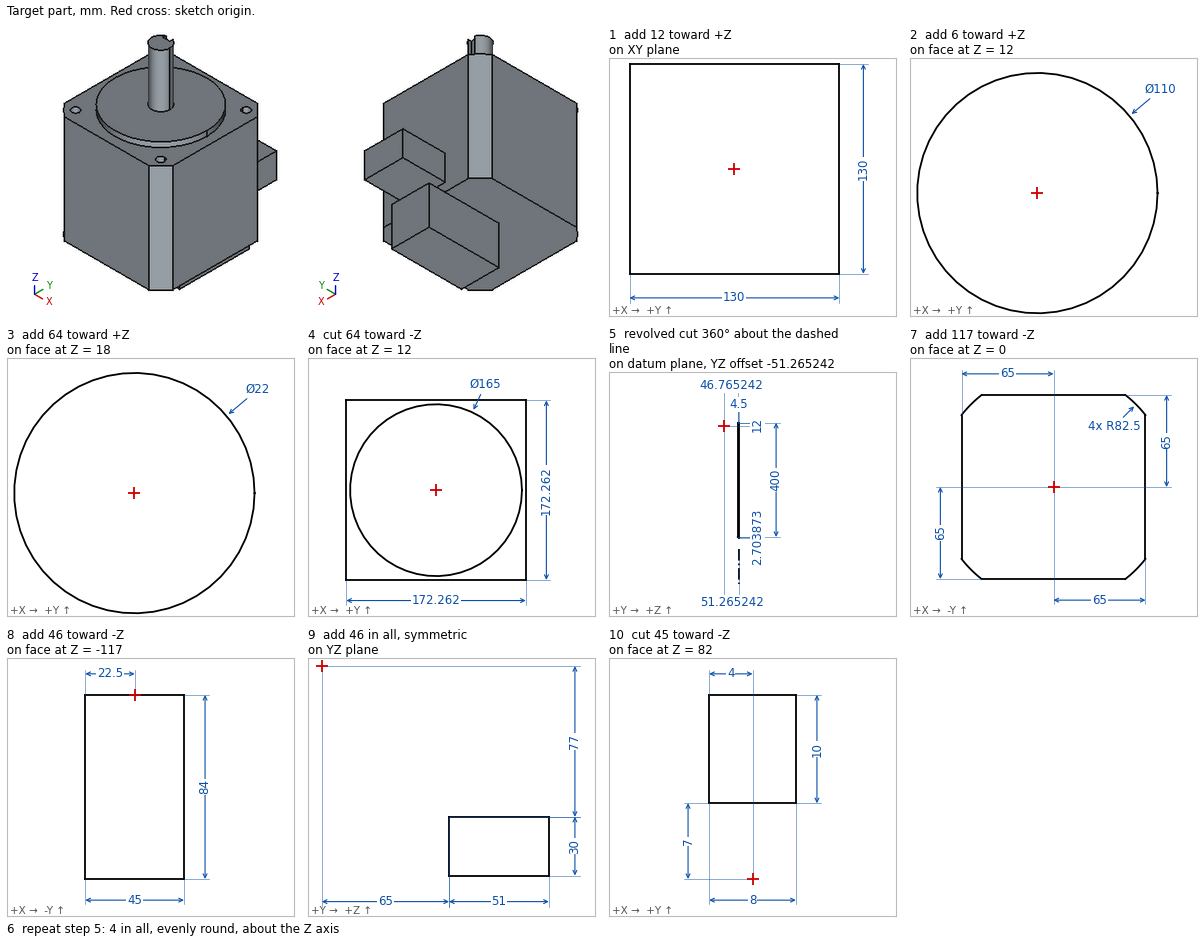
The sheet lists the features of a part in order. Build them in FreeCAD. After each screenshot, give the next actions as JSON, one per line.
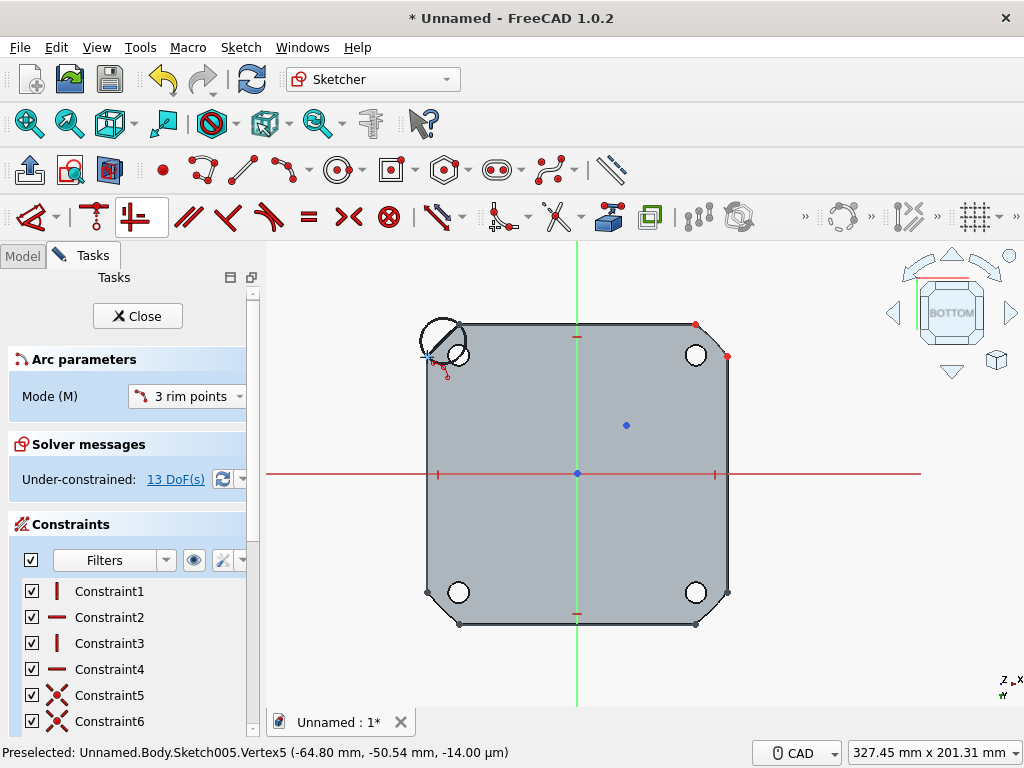
{"action": "scroll", "coordinate": [442, 339], "scroll_direction": "up", "scroll_amount": 13}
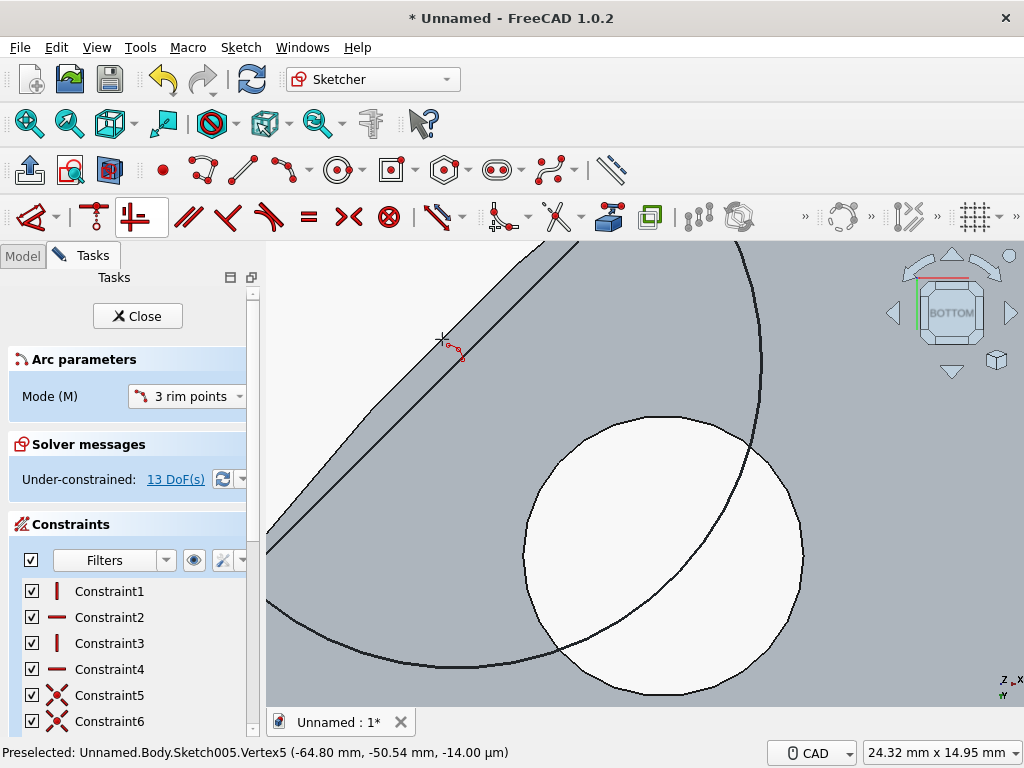
{"action": "left_click", "coordinate": [443, 336]}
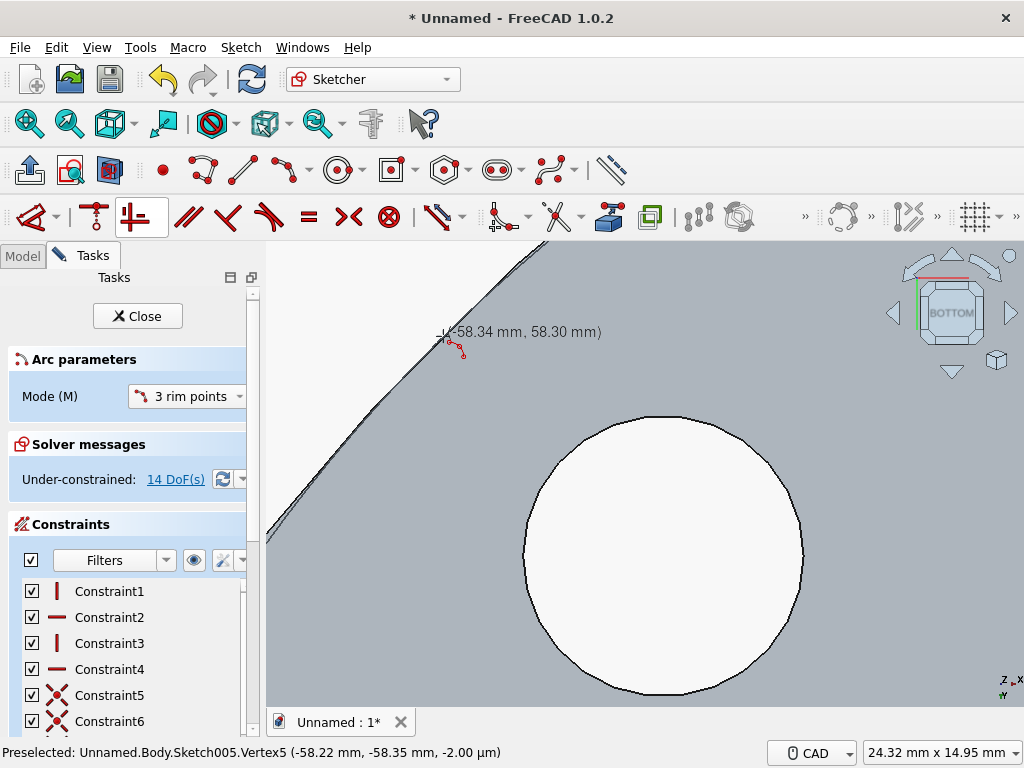
{"action": "scroll", "coordinate": [441, 339], "scroll_direction": "down", "scroll_amount": 13}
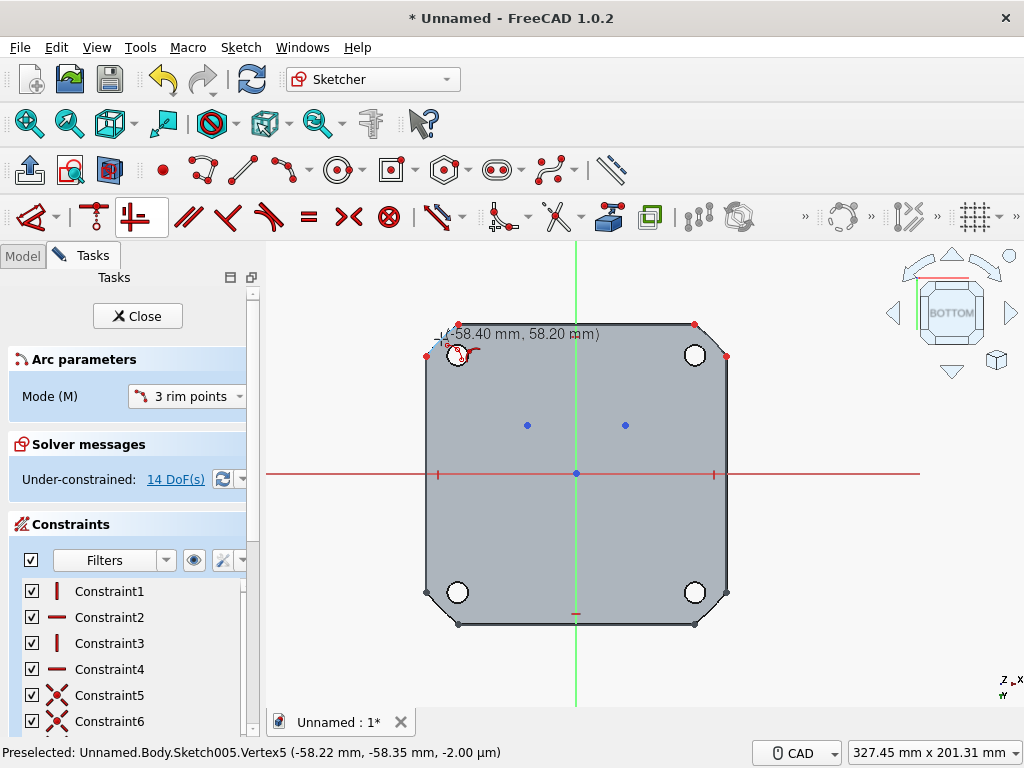
{"action": "left_click", "coordinate": [426, 593]}
{"action": "left_click", "coordinate": [458, 625]}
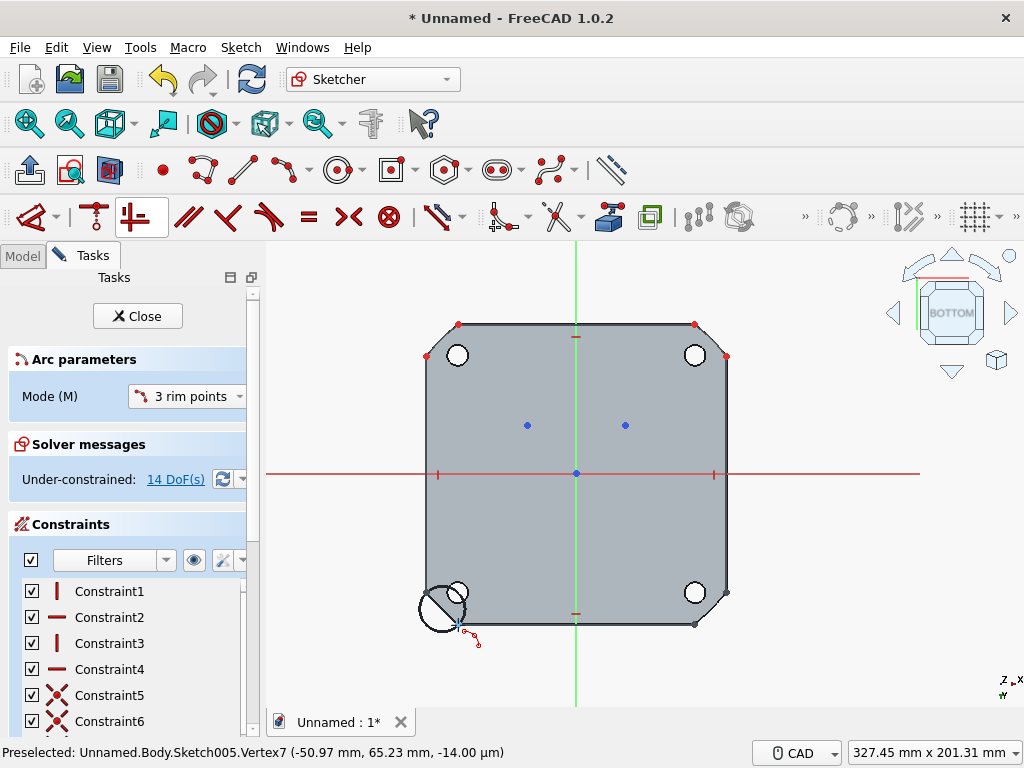
{"action": "scroll", "coordinate": [441, 609], "scroll_direction": "up", "scroll_amount": 13}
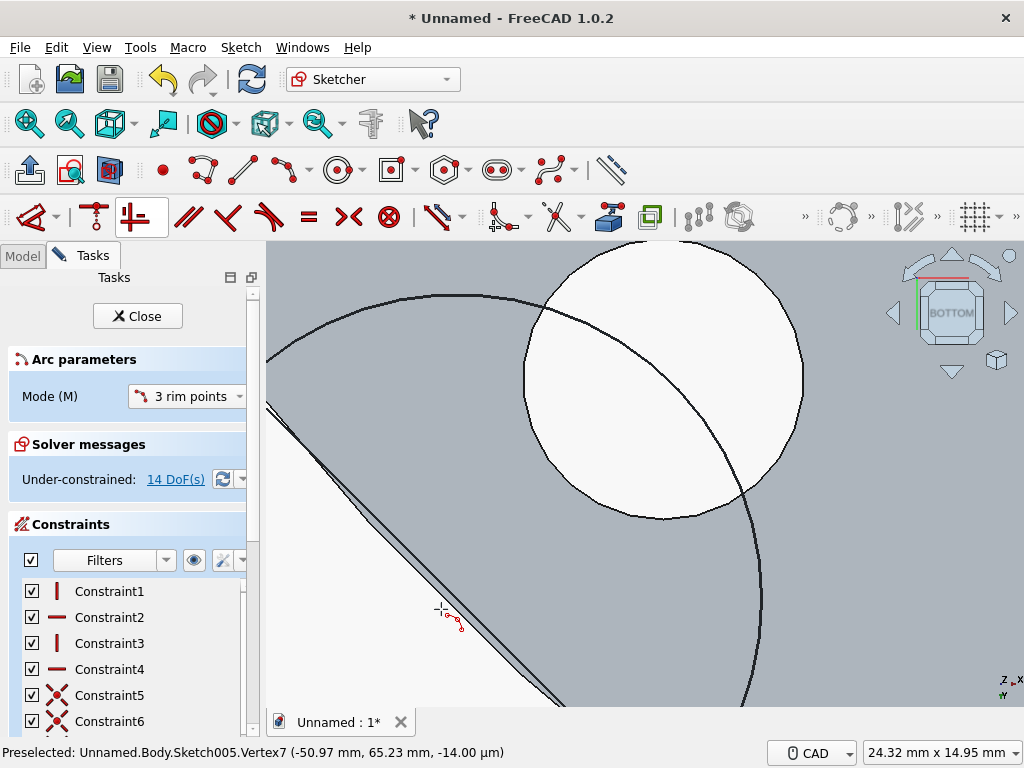
{"action": "left_click", "coordinate": [443, 600]}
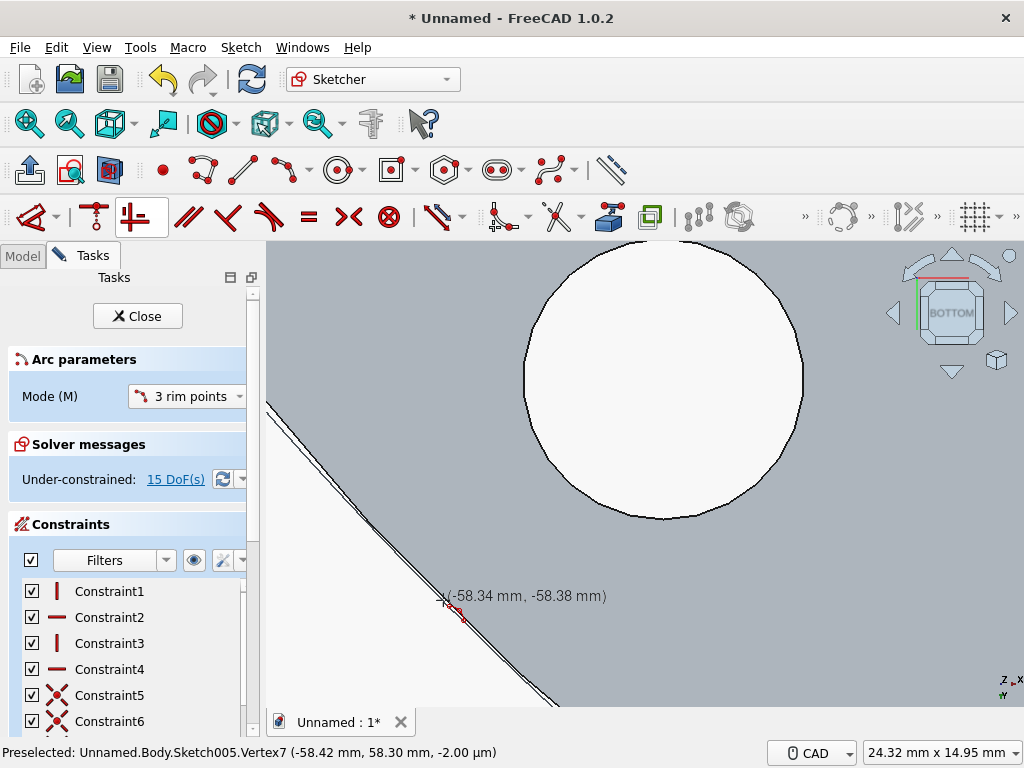
{"action": "scroll", "coordinate": [441, 610], "scroll_direction": "down", "scroll_amount": 13}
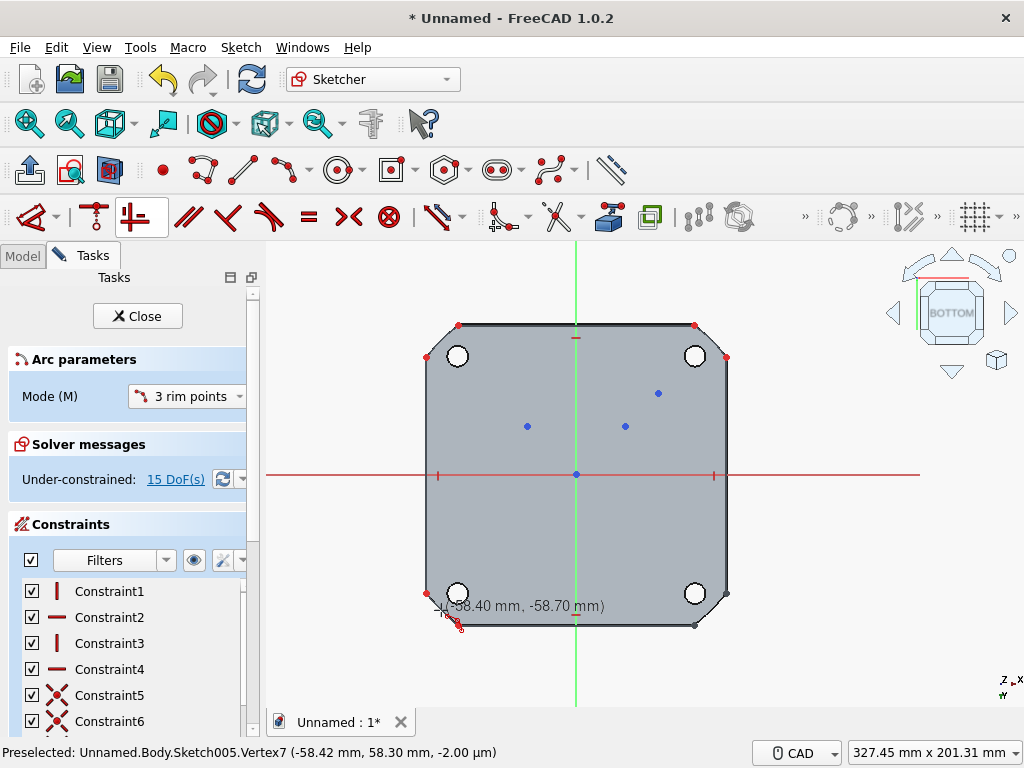
{"action": "left_click", "coordinate": [694, 626]}
{"action": "left_click", "coordinate": [726, 594]}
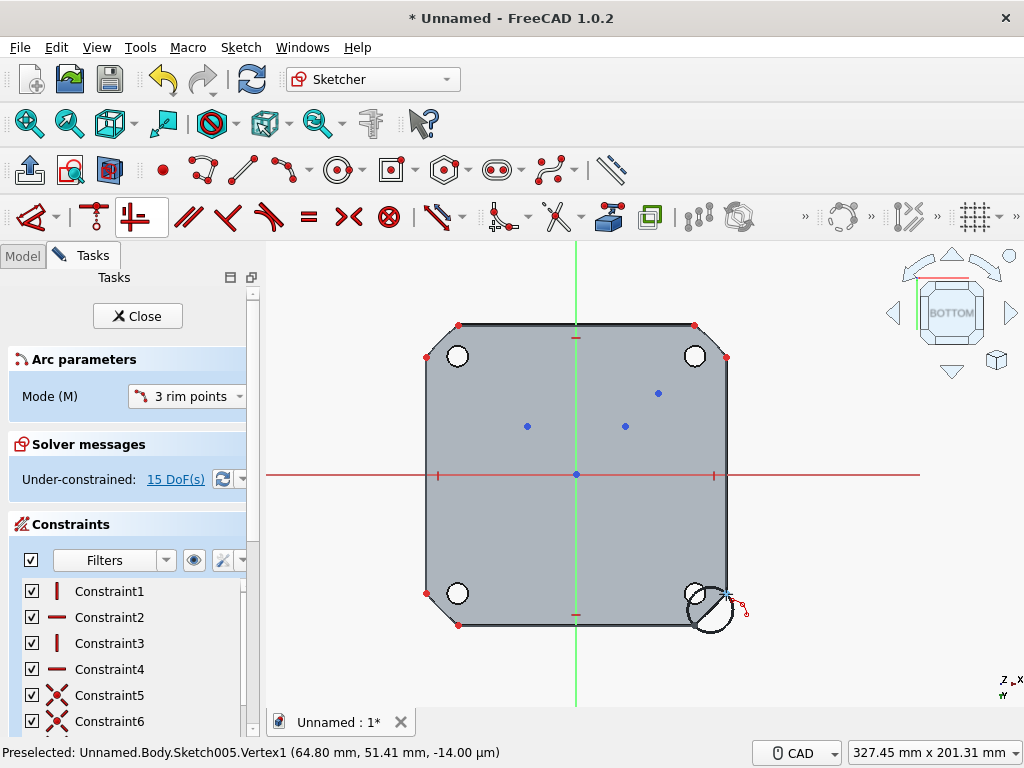
{"action": "scroll", "coordinate": [711, 610], "scroll_direction": "up", "scroll_amount": 13}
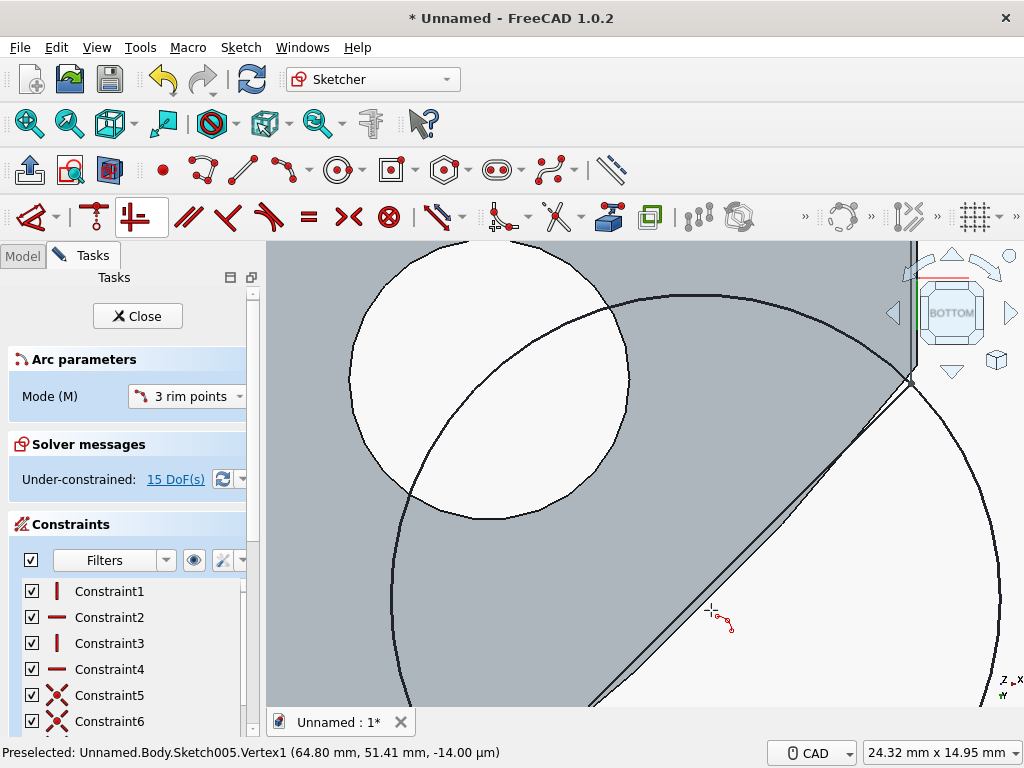
{"action": "left_click", "coordinate": [710, 600]}
{"action": "key", "text": "Escape"}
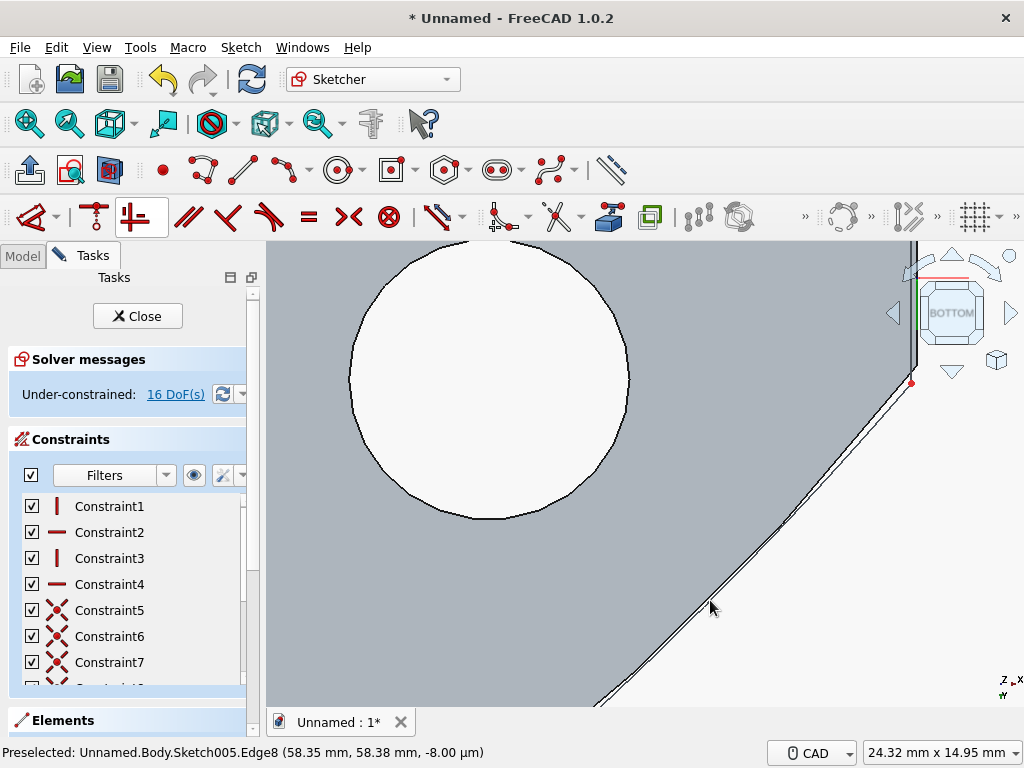
{"action": "scroll", "coordinate": [712, 610], "scroll_direction": "down", "scroll_amount": 13}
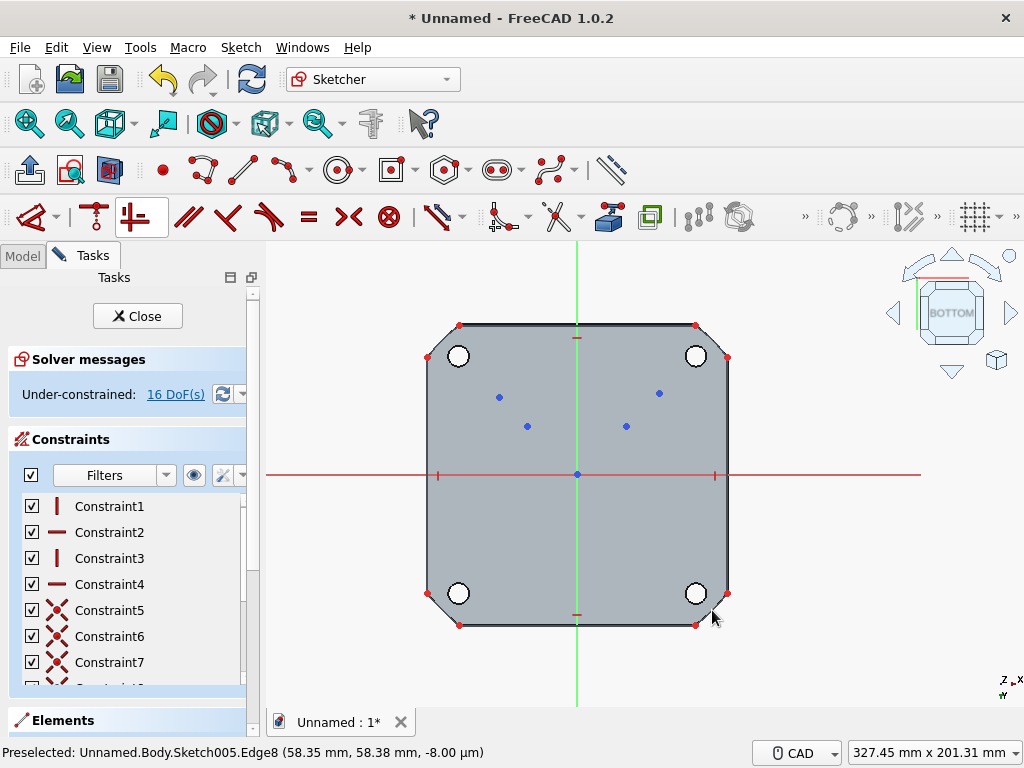
{"action": "left_click", "coordinate": [719, 347]}